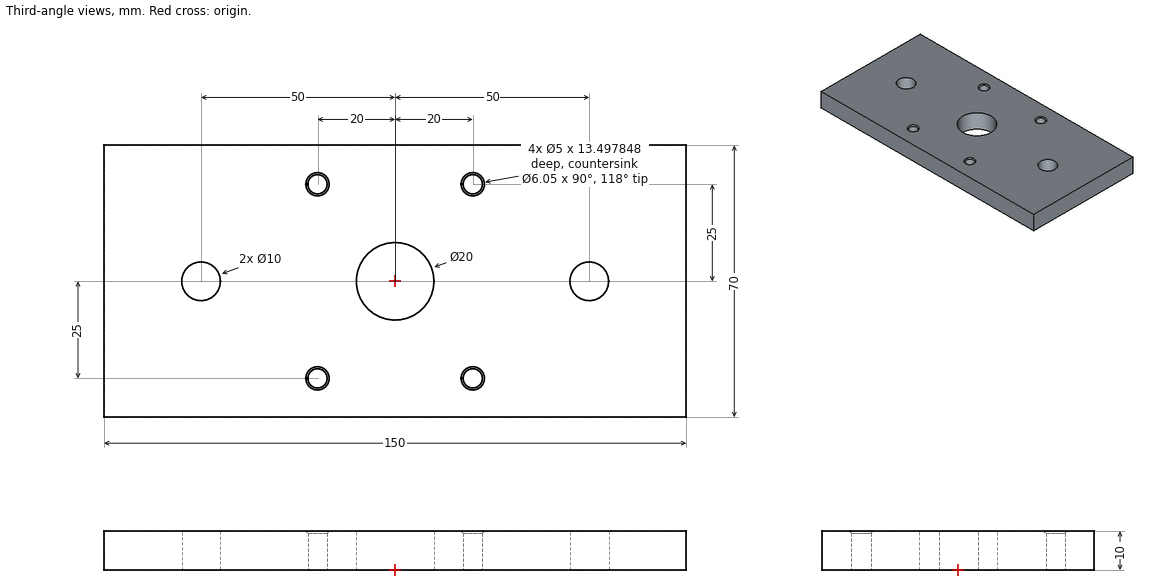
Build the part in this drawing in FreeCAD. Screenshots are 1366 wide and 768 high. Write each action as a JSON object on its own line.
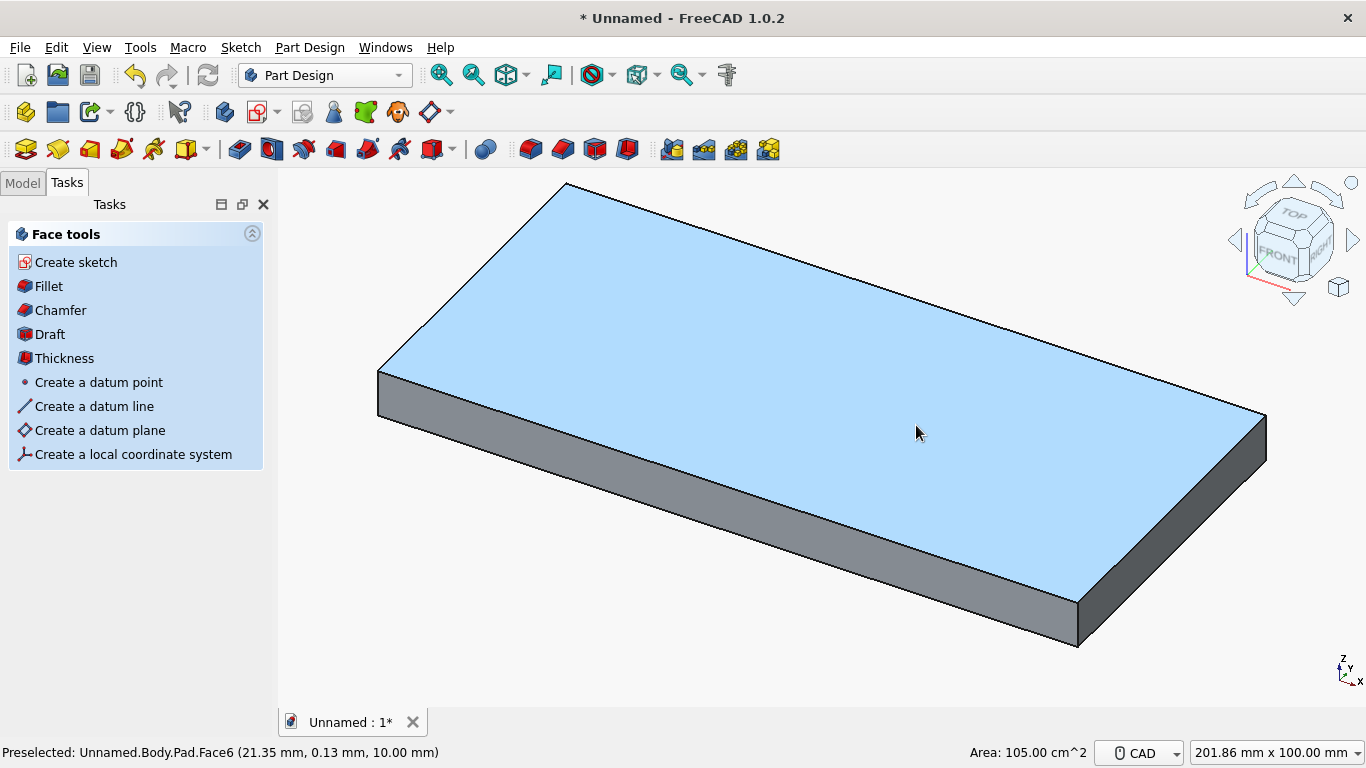
{"action": "left_click", "coordinate": [258, 112]}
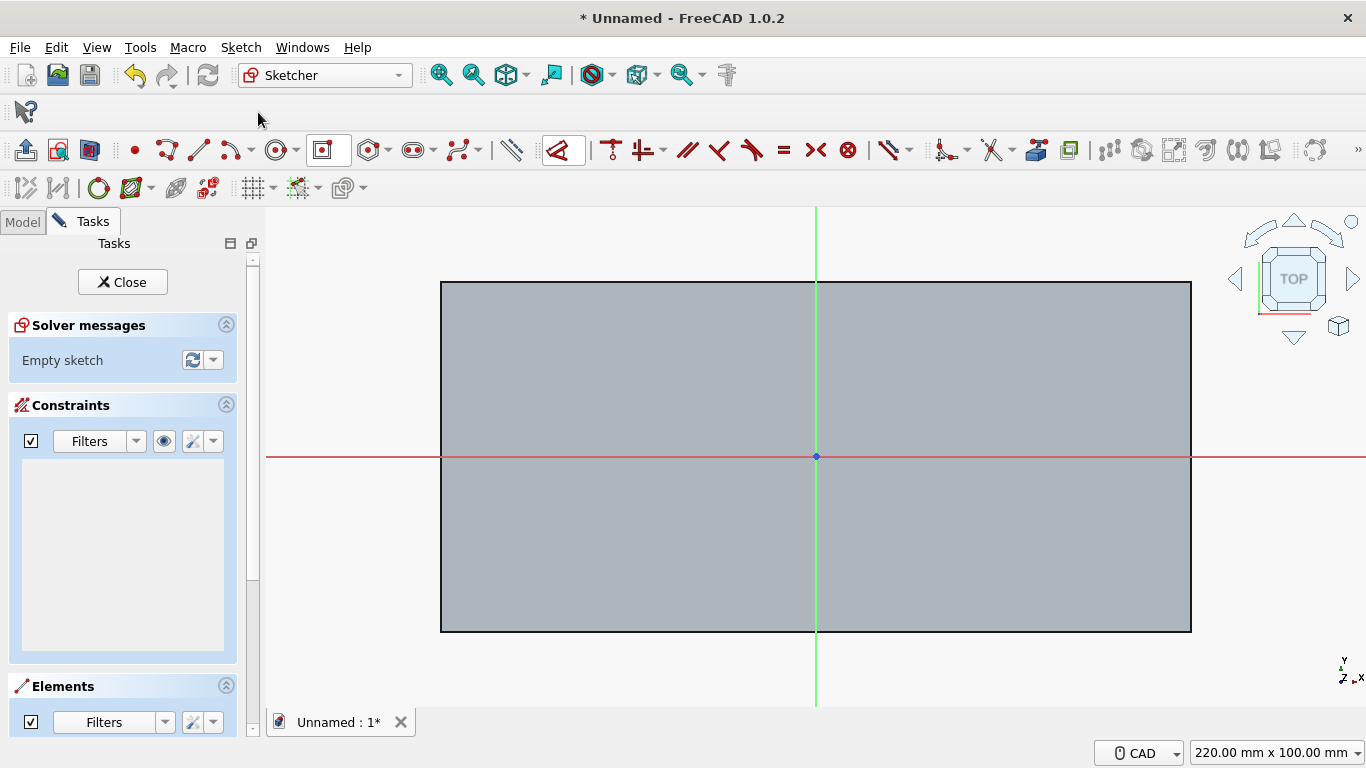
{"action": "scroll", "coordinate": [846, 457], "scroll_direction": "up", "scroll_amount": 6}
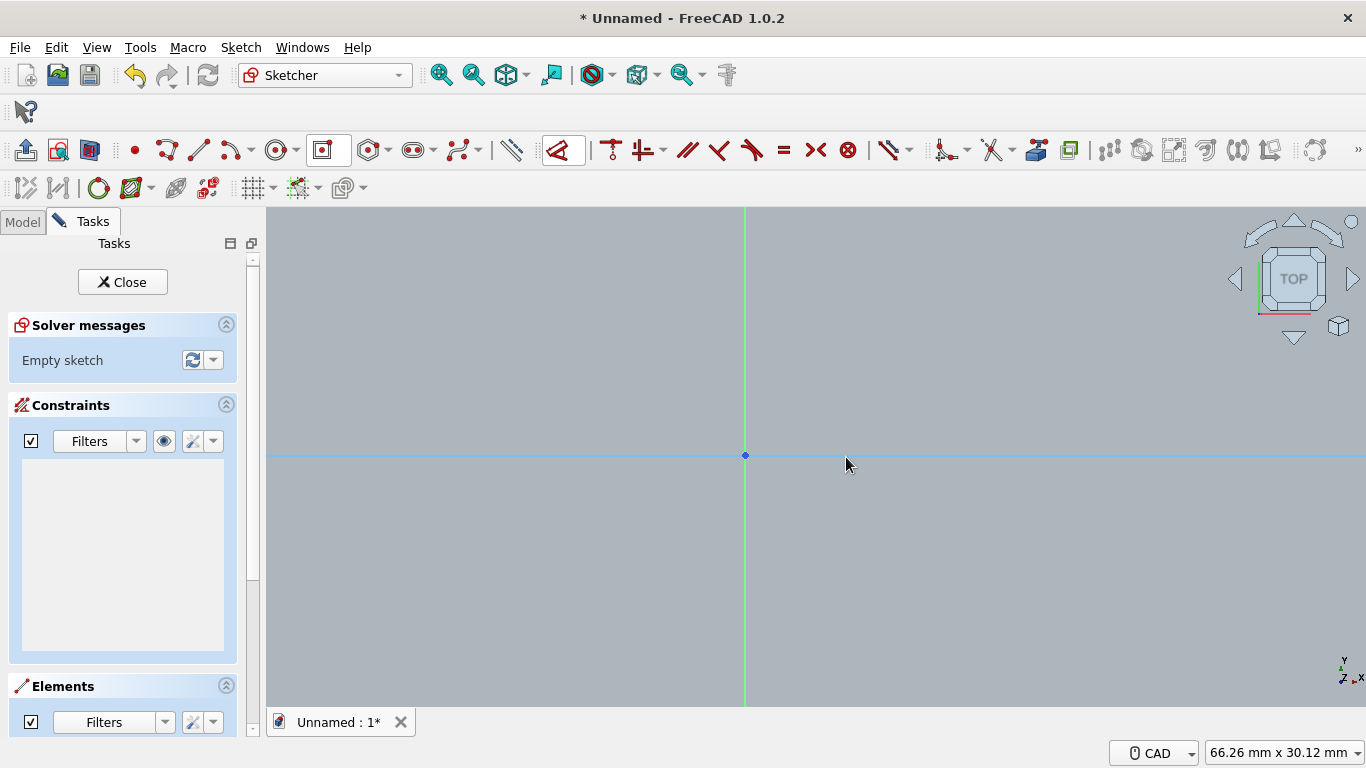
{"action": "left_click", "coordinate": [276, 150]}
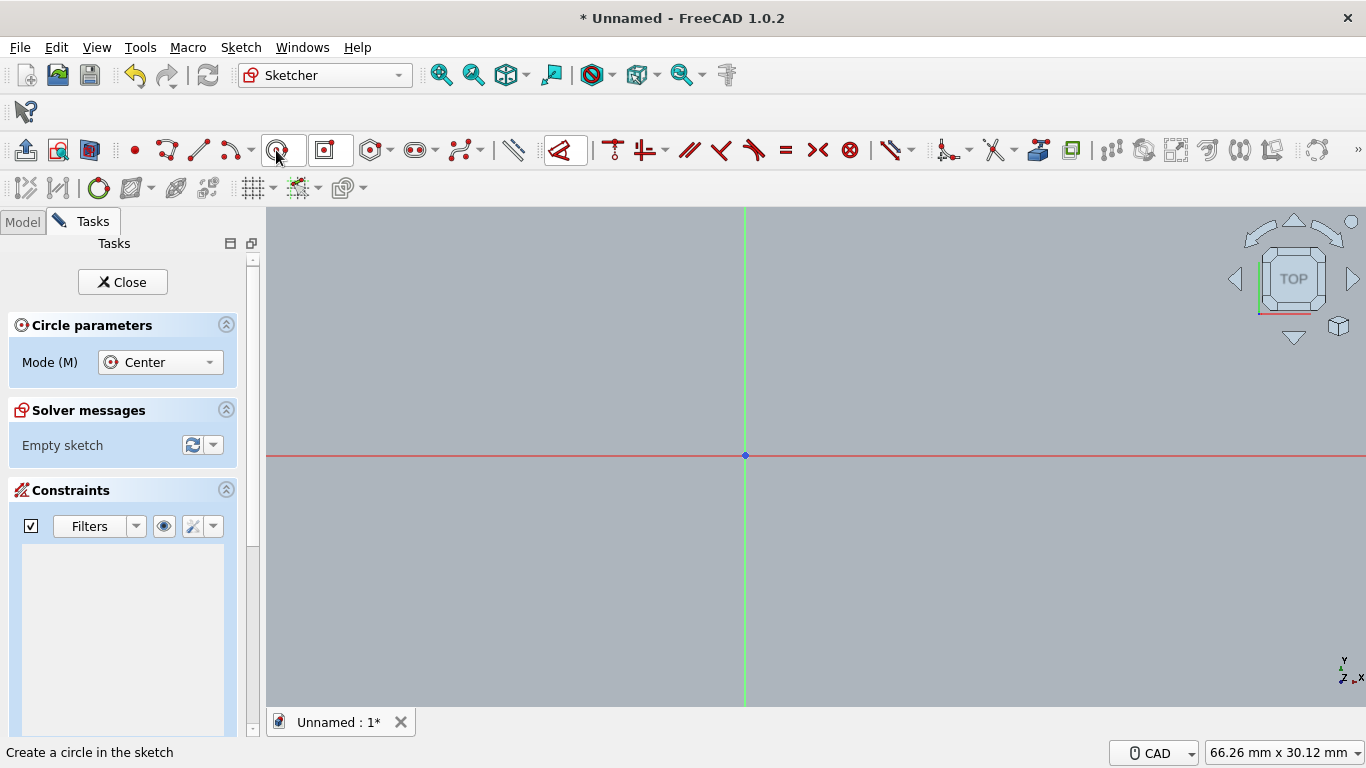
{"action": "left_click", "coordinate": [745, 456]}
{"action": "left_click", "coordinate": [863, 338]}
{"action": "key", "text": "Escape"}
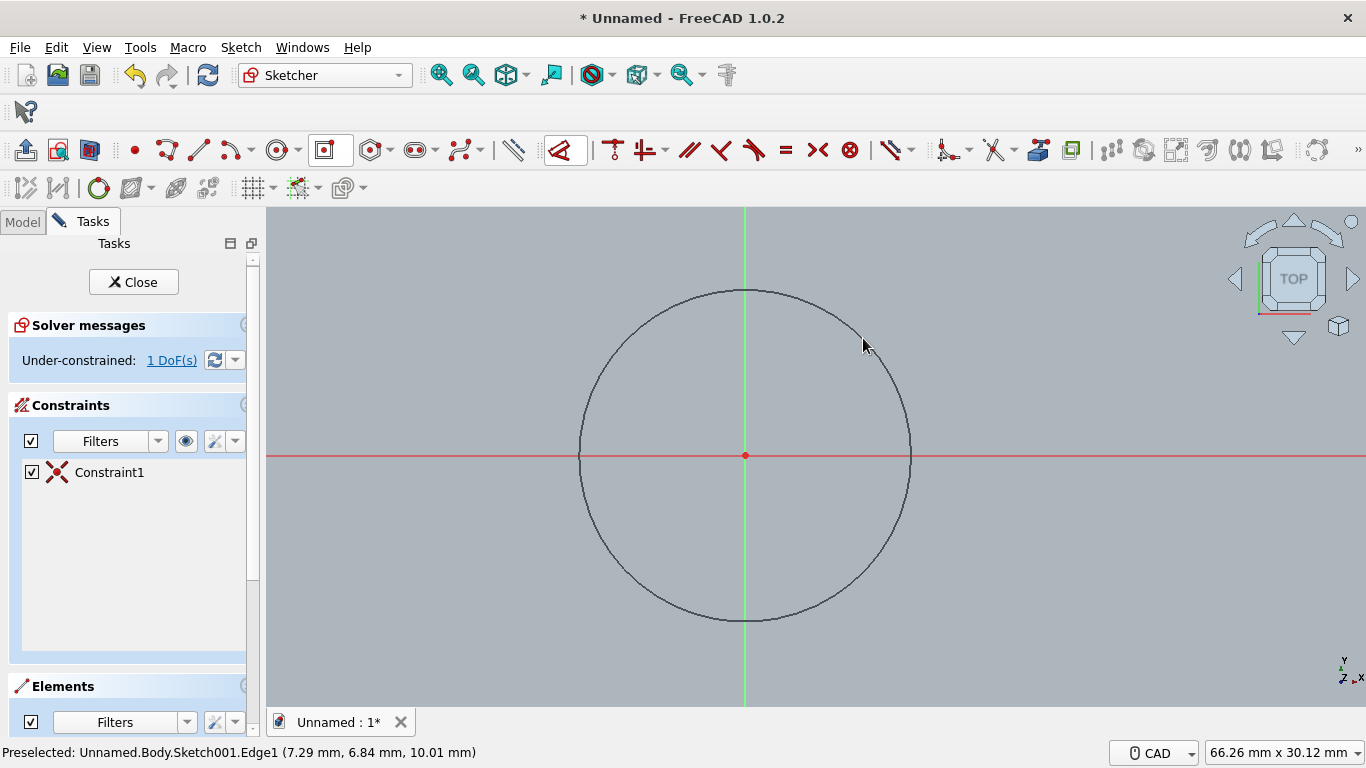
{"action": "left_click", "coordinate": [862, 338]}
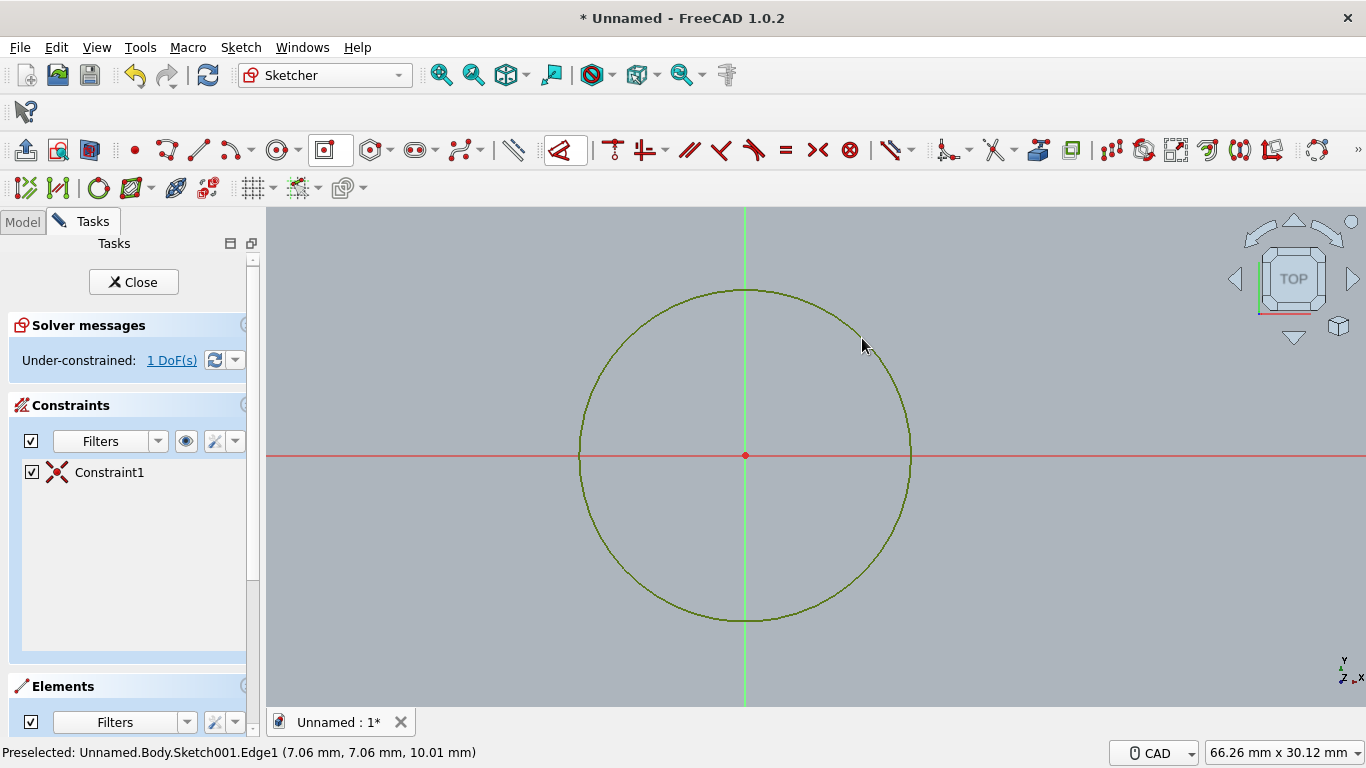
{"action": "left_click", "coordinate": [582, 150]}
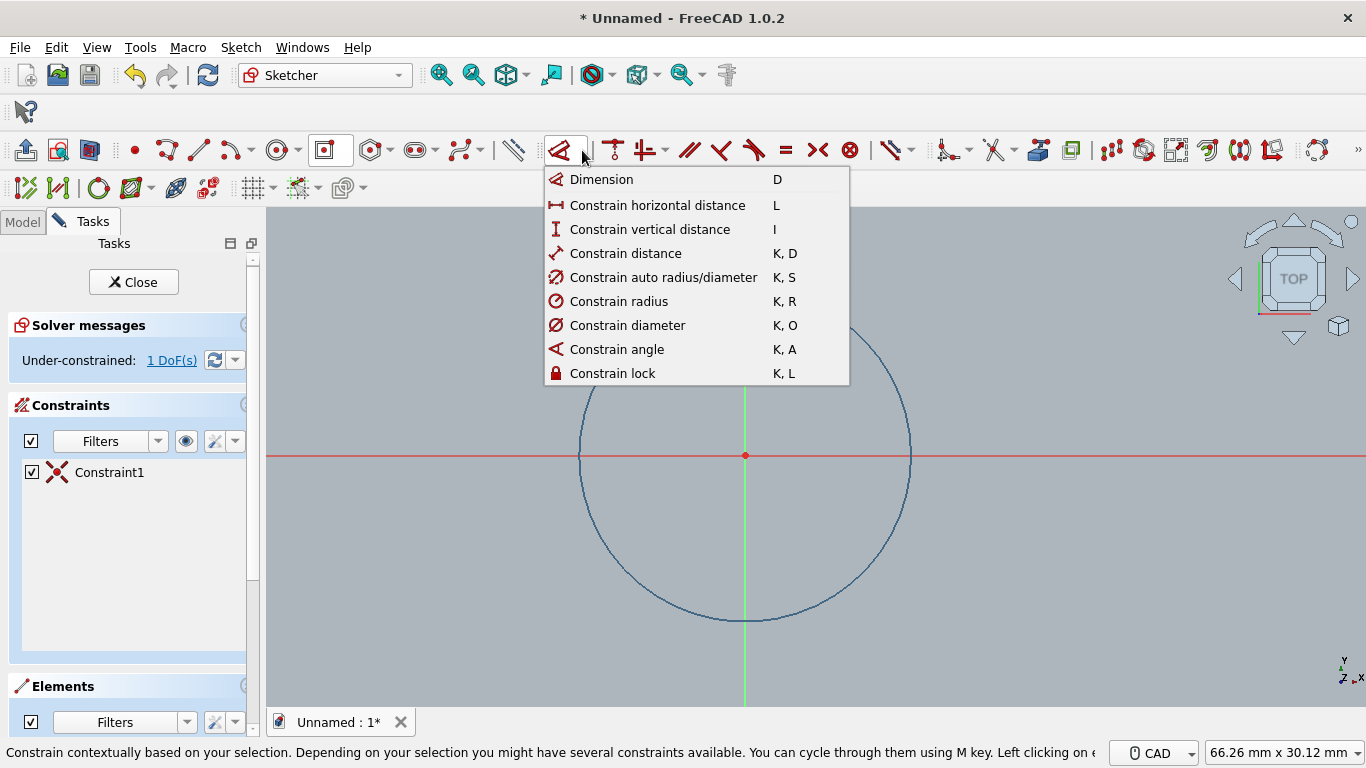
{"action": "left_click", "coordinate": [697, 325]}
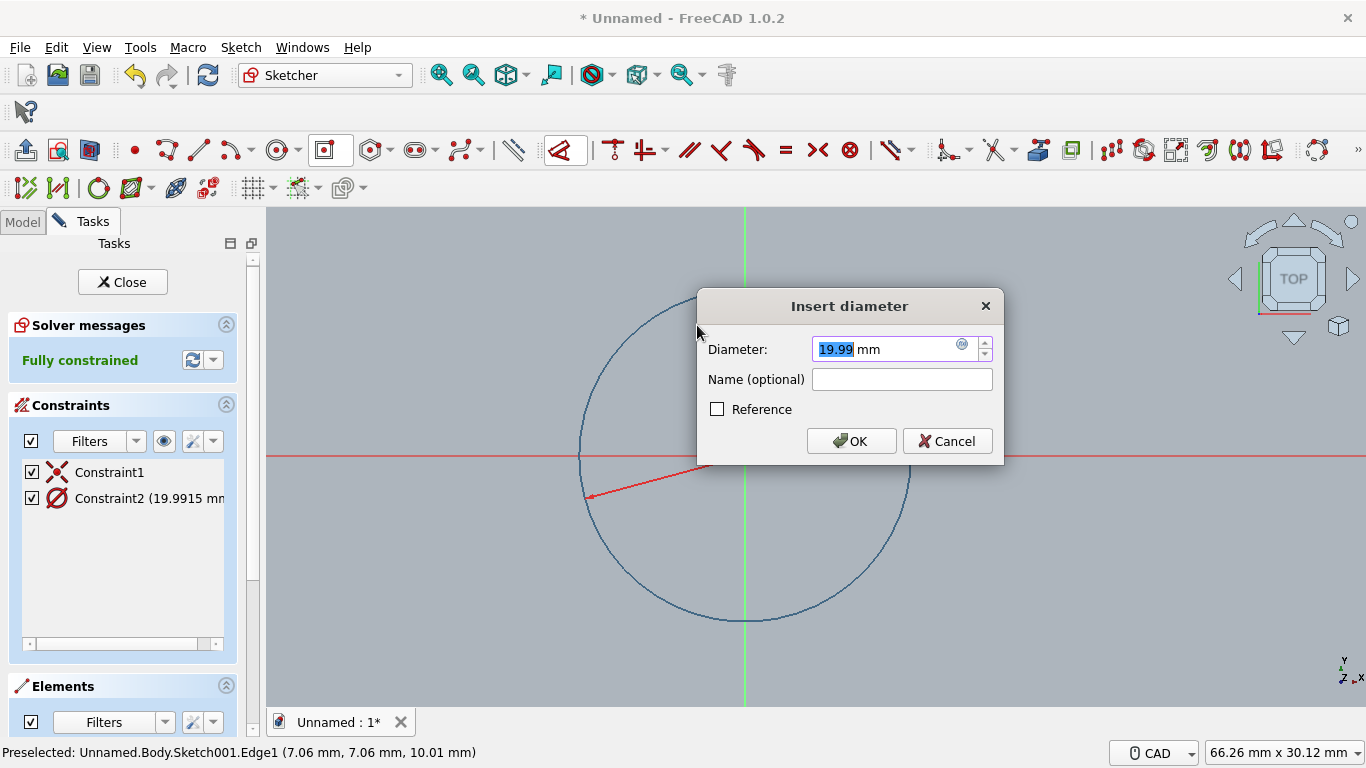
{"action": "type", "text": "20"}
{"action": "key", "text": "Return"}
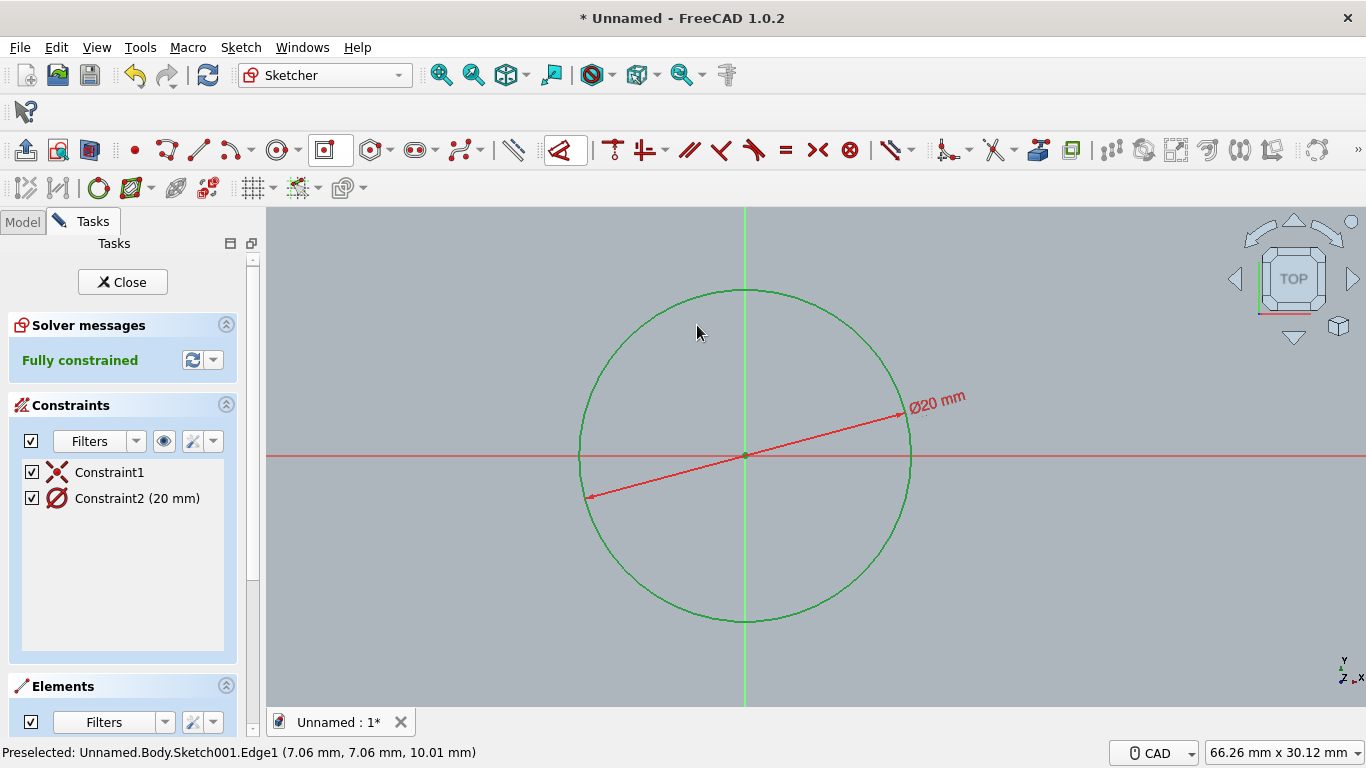
{"action": "left_click", "coordinate": [123, 282]}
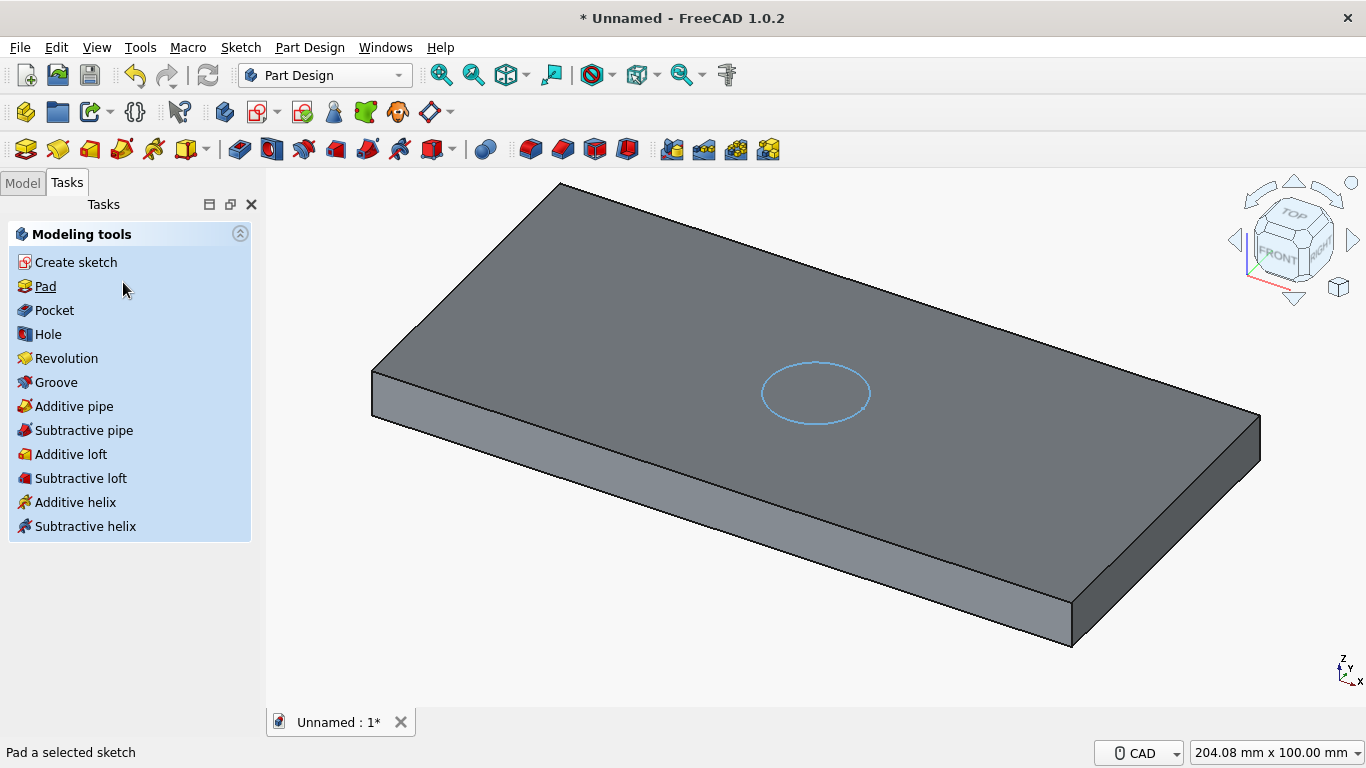
{"action": "left_click", "coordinate": [240, 150]}